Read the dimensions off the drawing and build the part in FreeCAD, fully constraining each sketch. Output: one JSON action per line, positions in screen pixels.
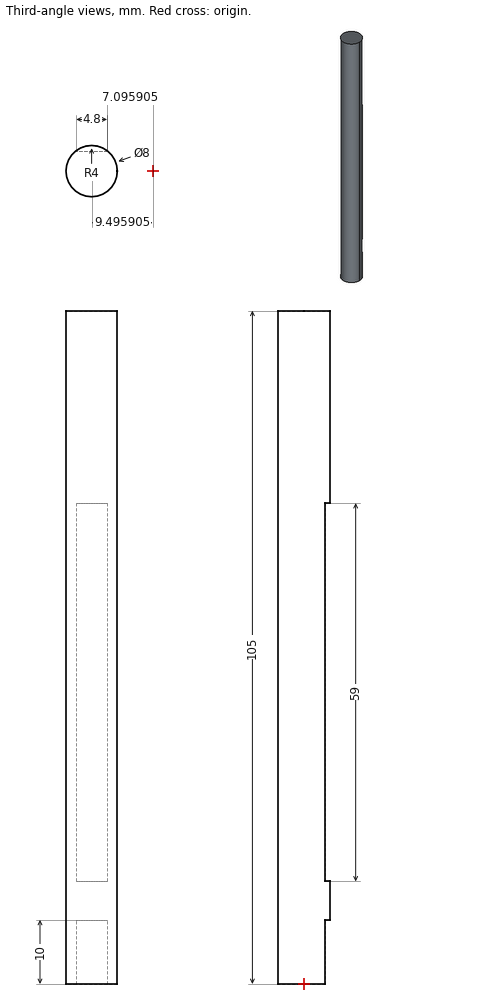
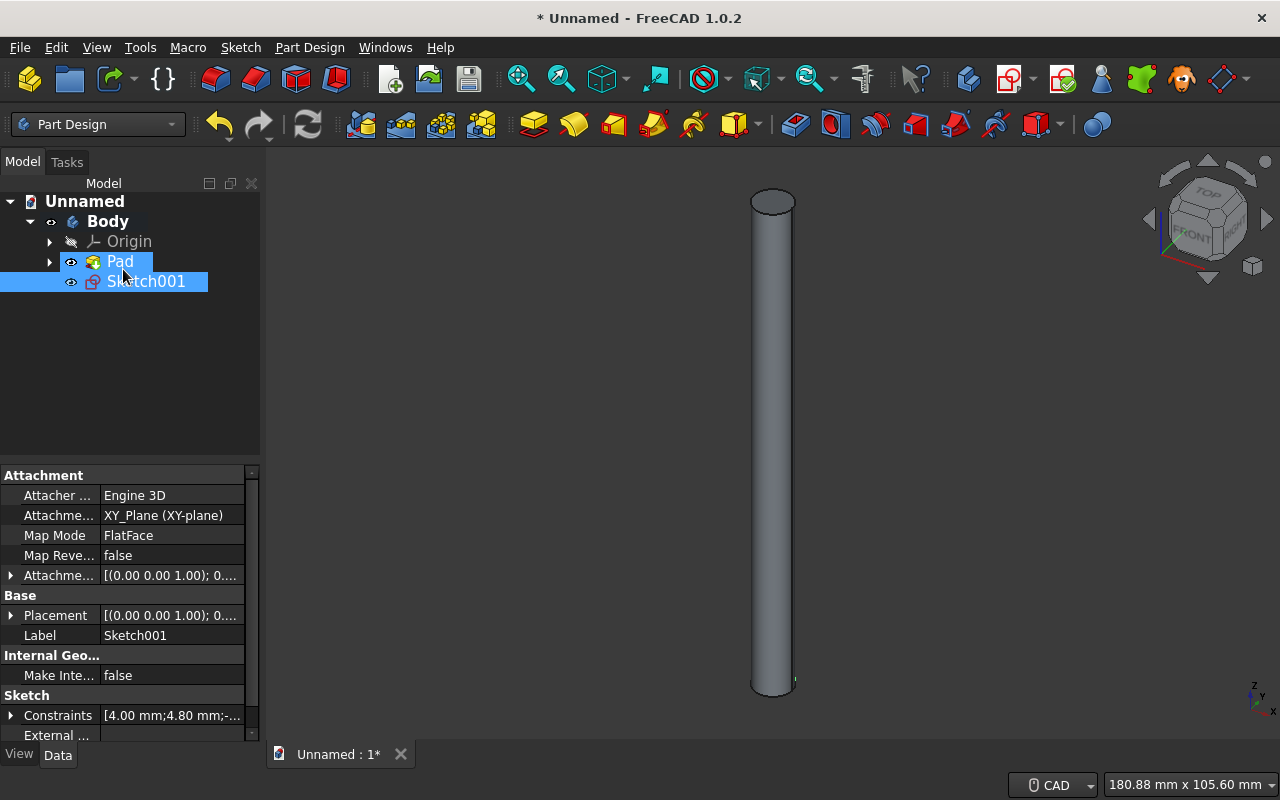
{"action": "left_click", "coordinate": [796, 124]}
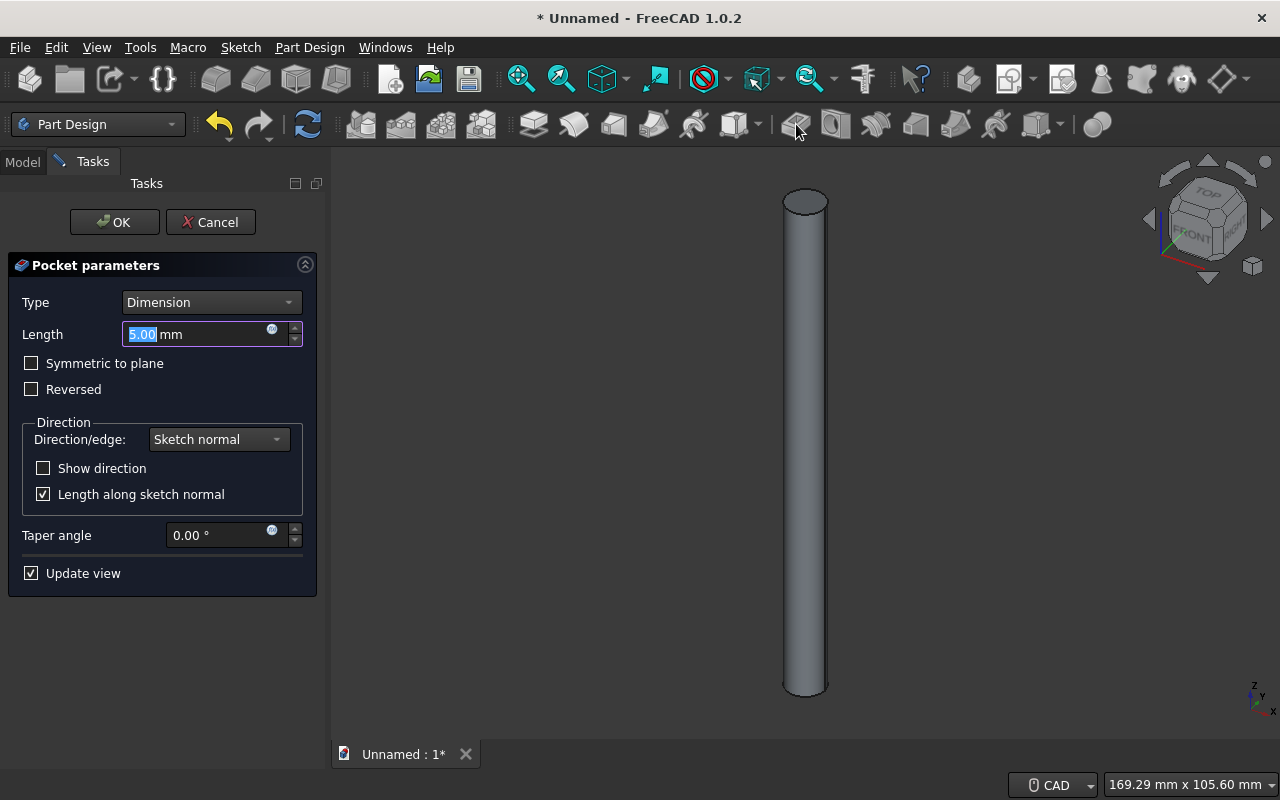
{"action": "type", "text": "10"}
{"action": "key", "text": "Tab"}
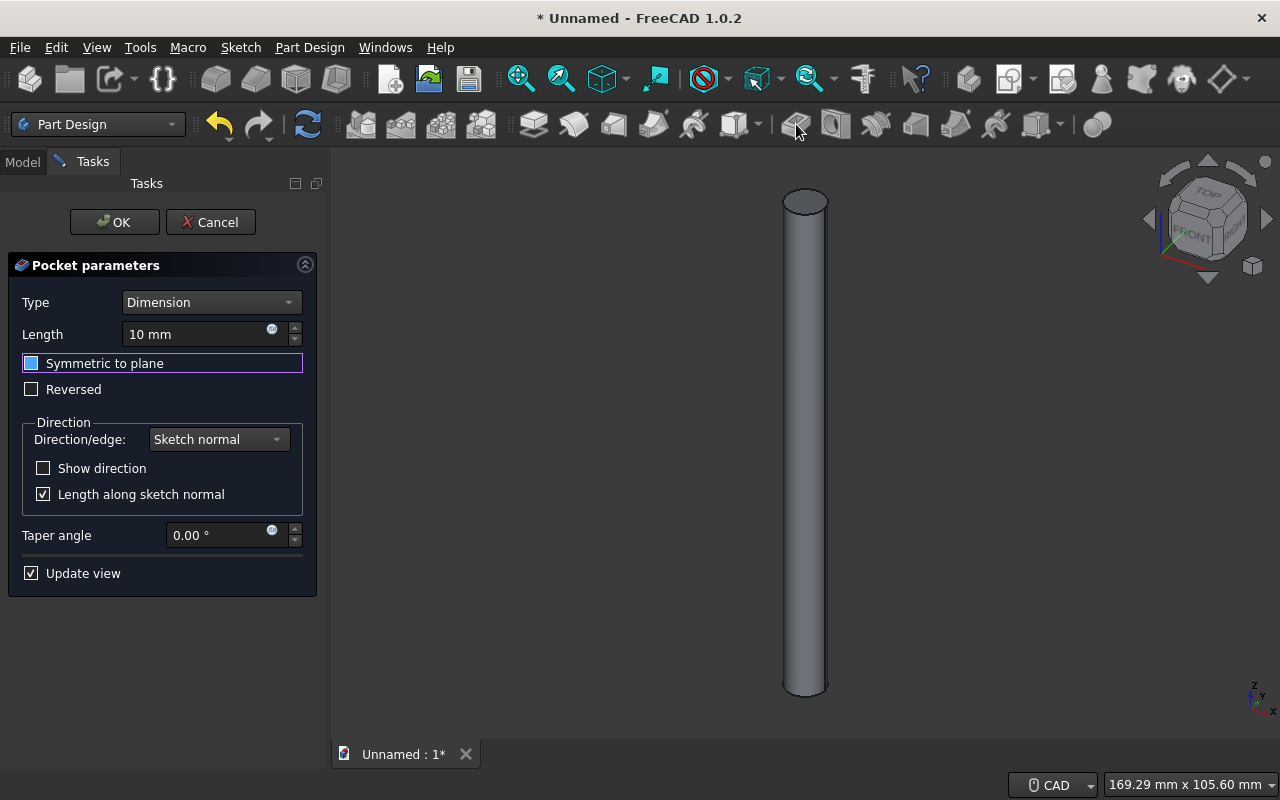
{"action": "left_click", "coordinate": [30, 389]}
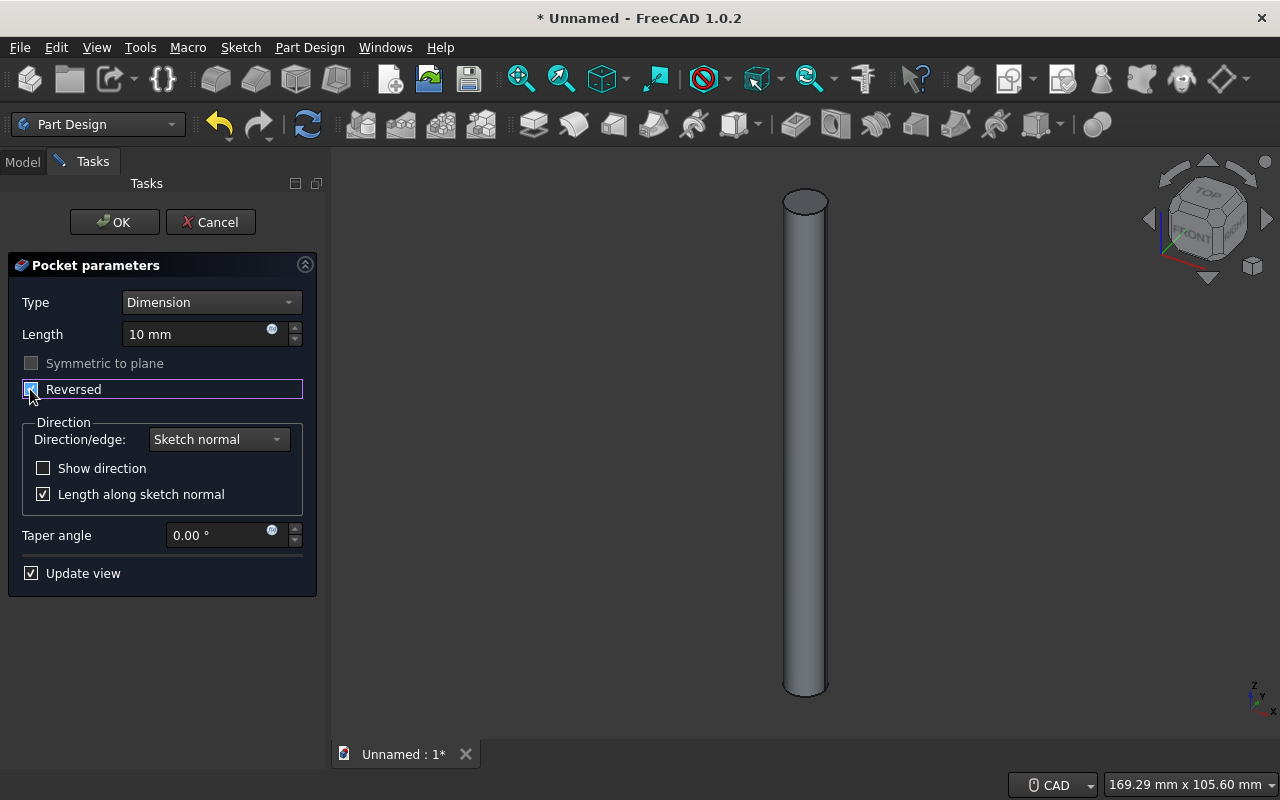
{"action": "left_click", "coordinate": [115, 222]}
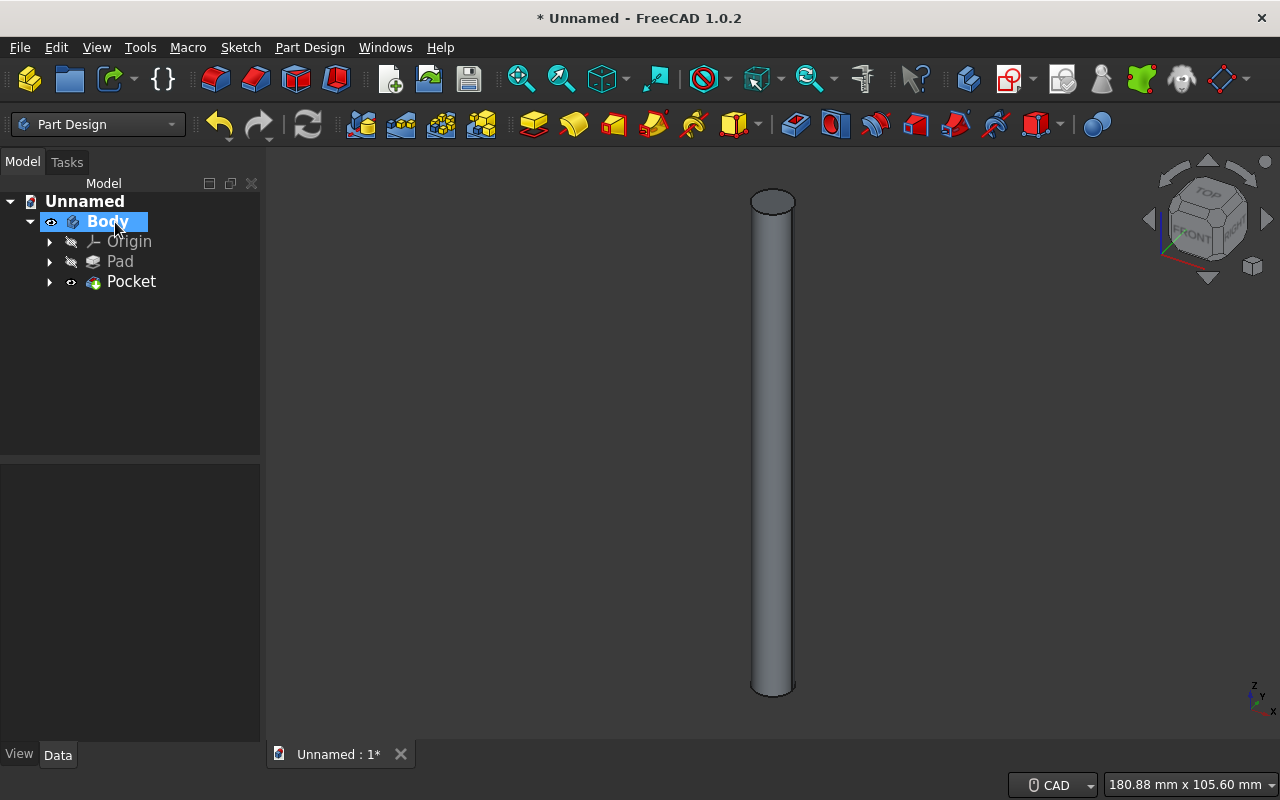
{"action": "left_click", "coordinate": [50, 242]}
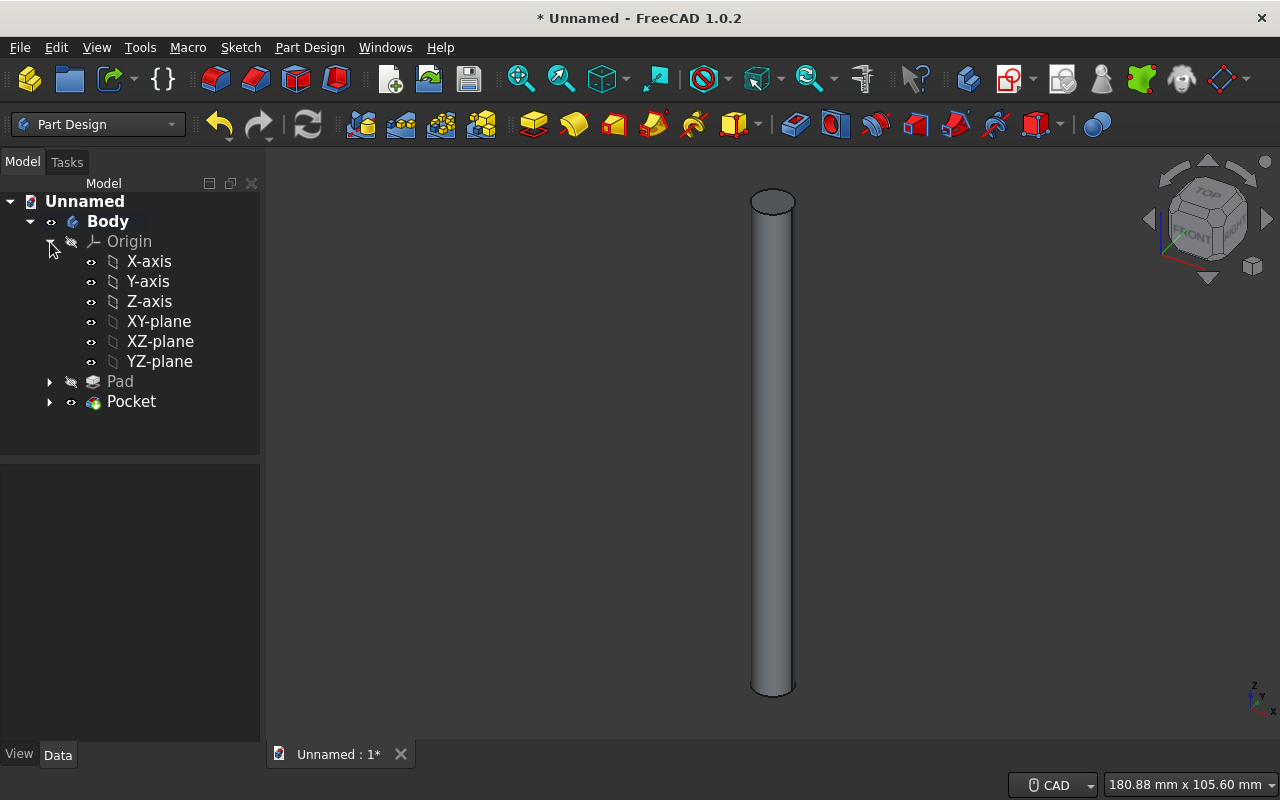
{"action": "left_click", "coordinate": [136, 322]}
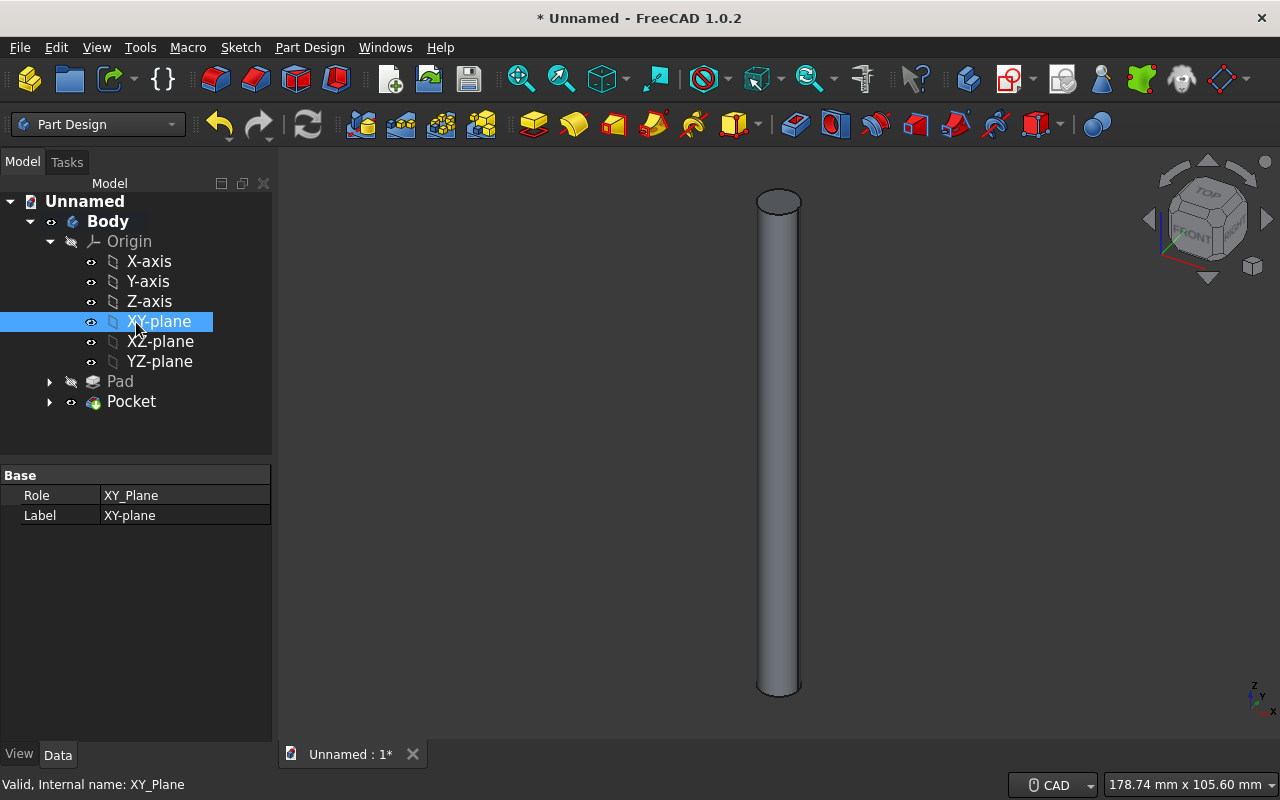
{"action": "left_click", "coordinate": [1222, 80]}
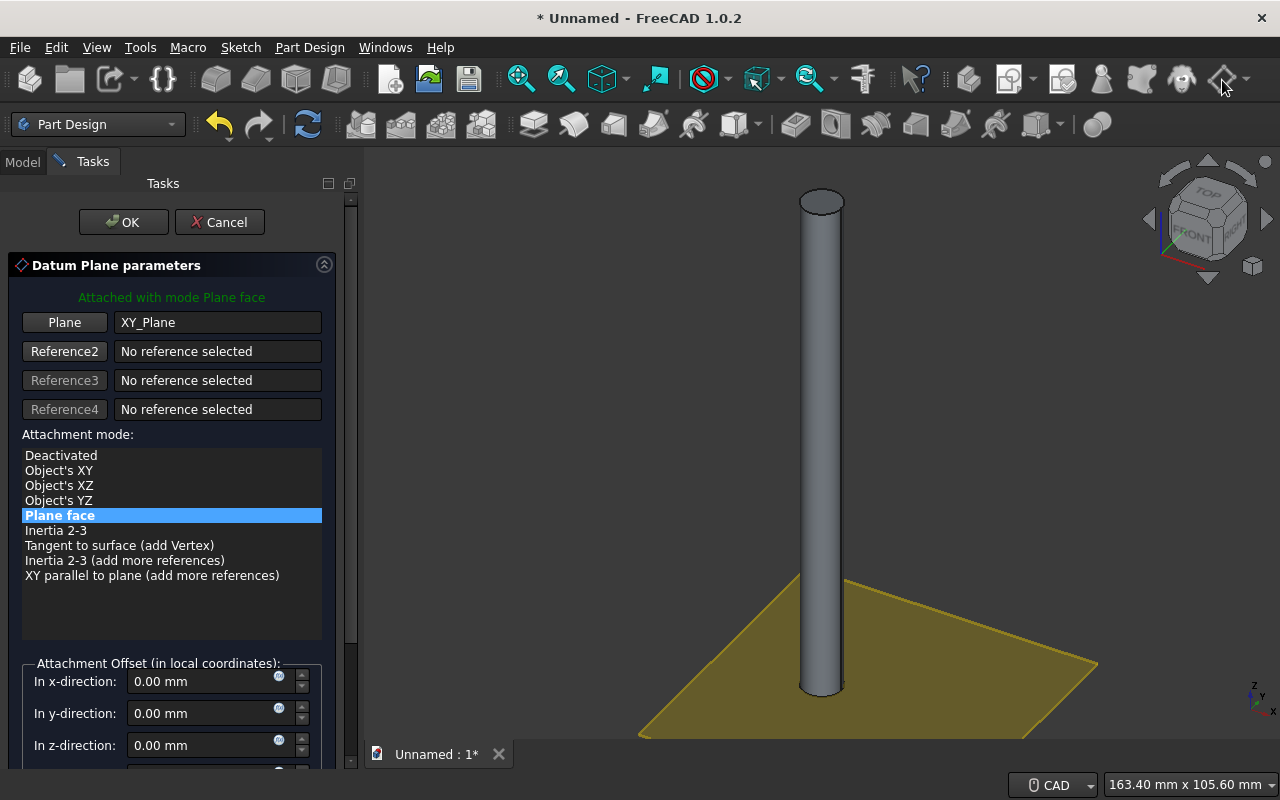
{"action": "triple_click", "coordinate": [210, 745]}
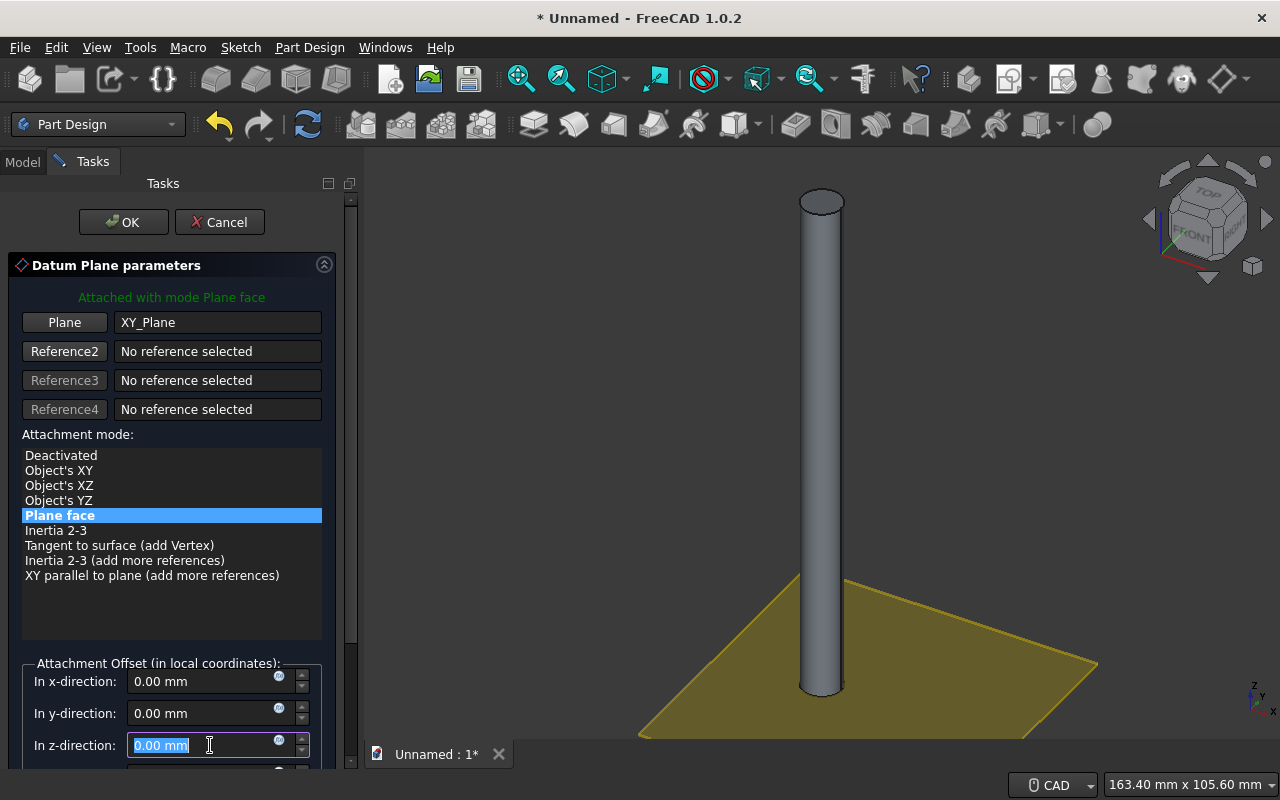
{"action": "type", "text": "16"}
{"action": "key", "text": "Tab"}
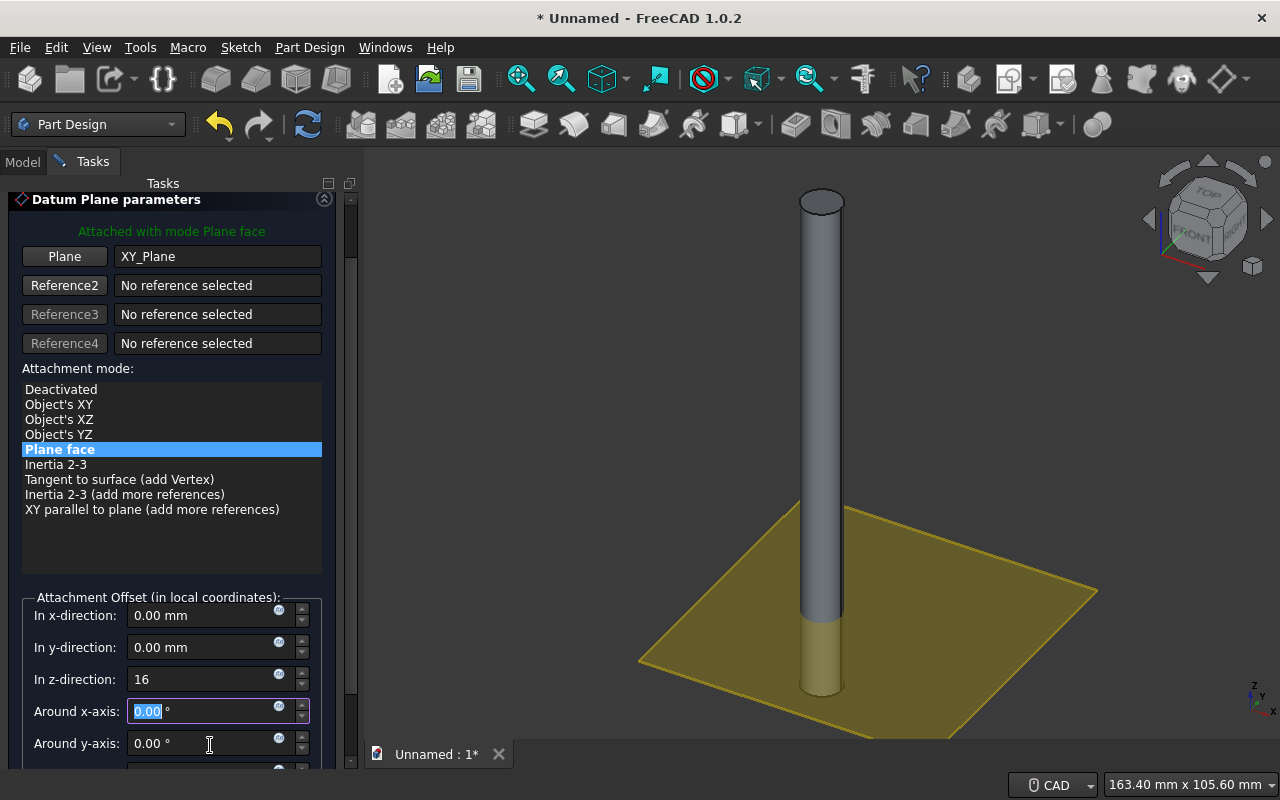
{"action": "scroll", "coordinate": [351, 480], "scroll_direction": "up", "scroll_amount": 2}